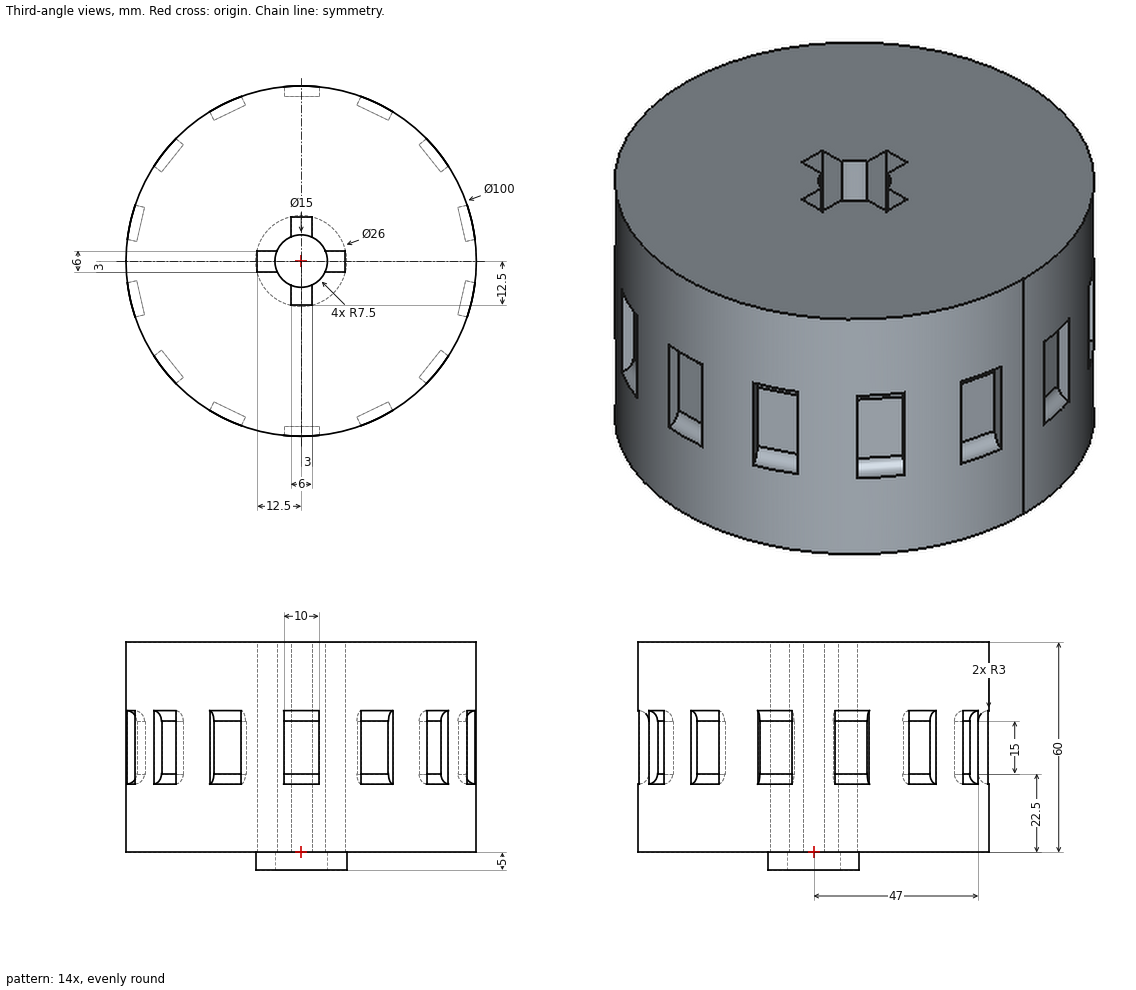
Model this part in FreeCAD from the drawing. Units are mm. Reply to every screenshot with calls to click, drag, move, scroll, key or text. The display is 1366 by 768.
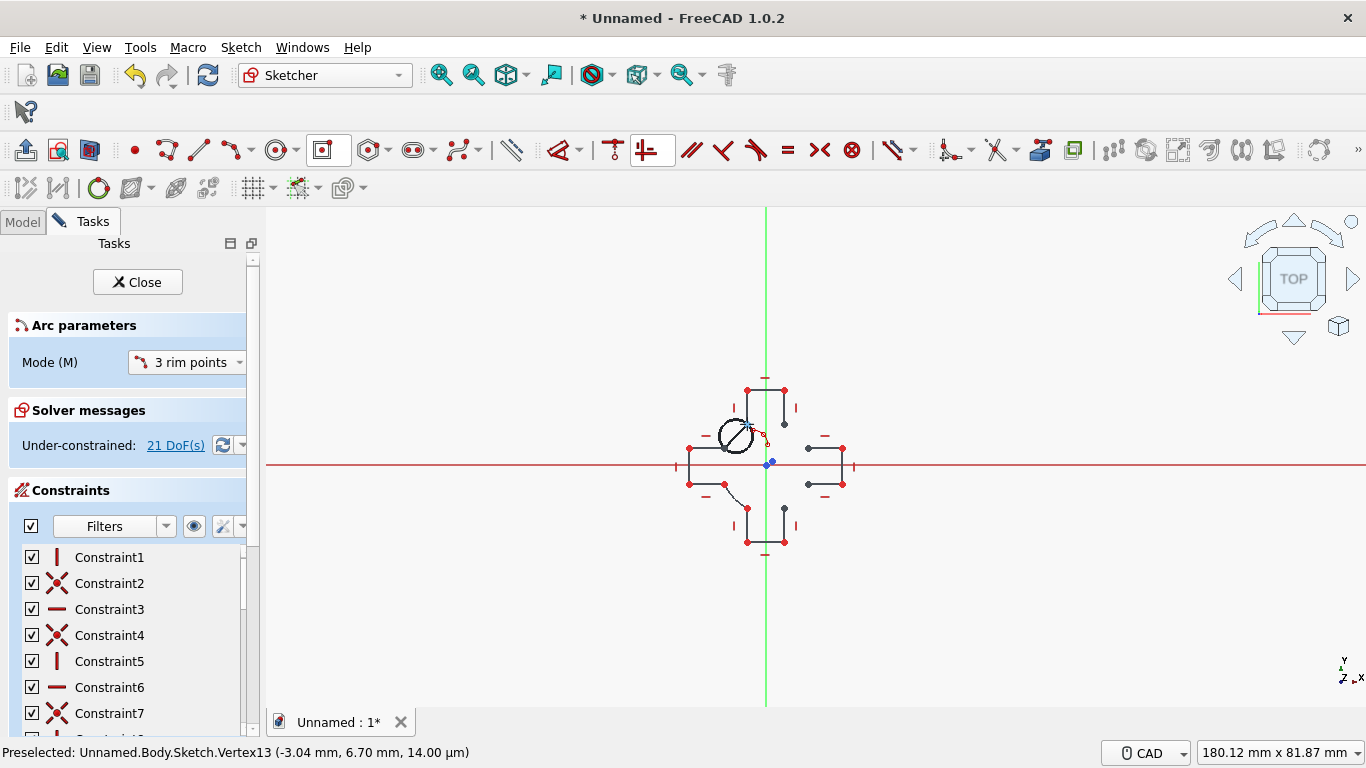
scroll(734, 433, up, 9)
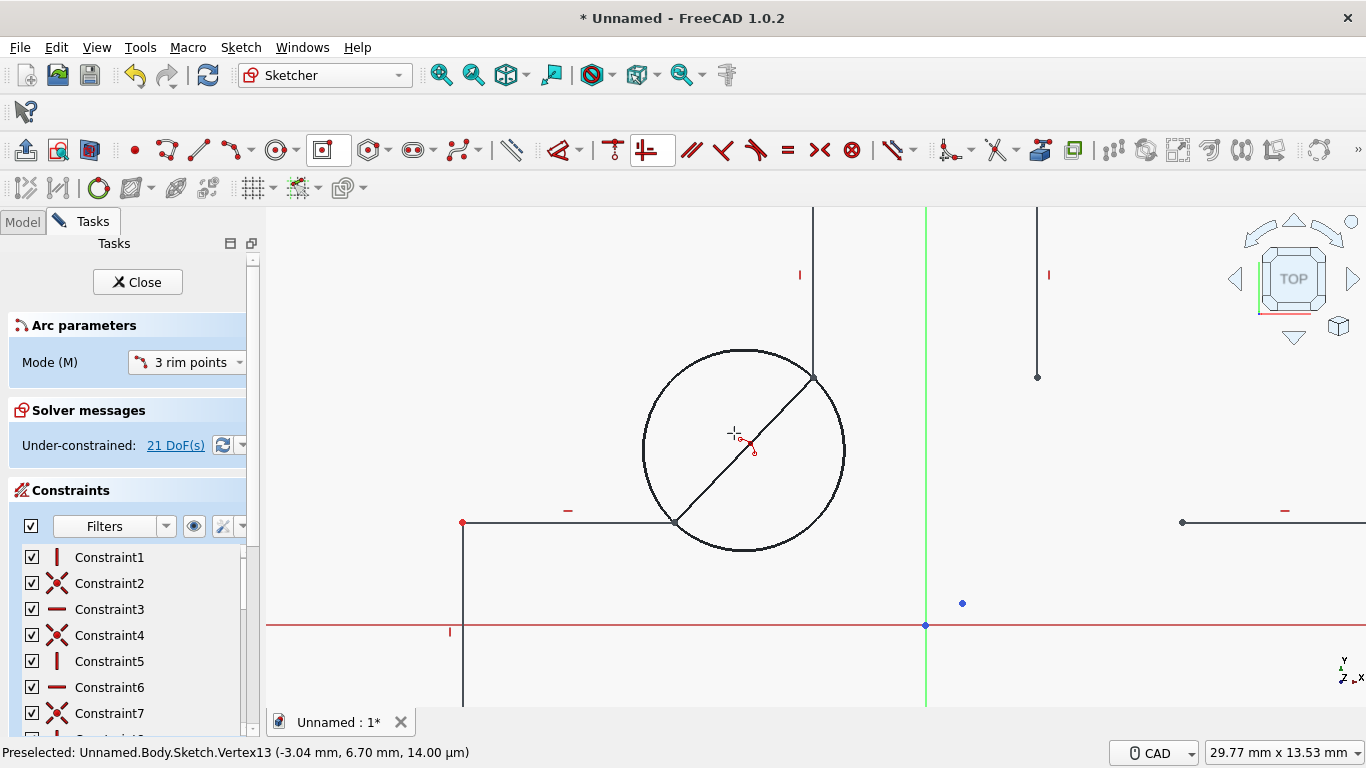
click(730, 430)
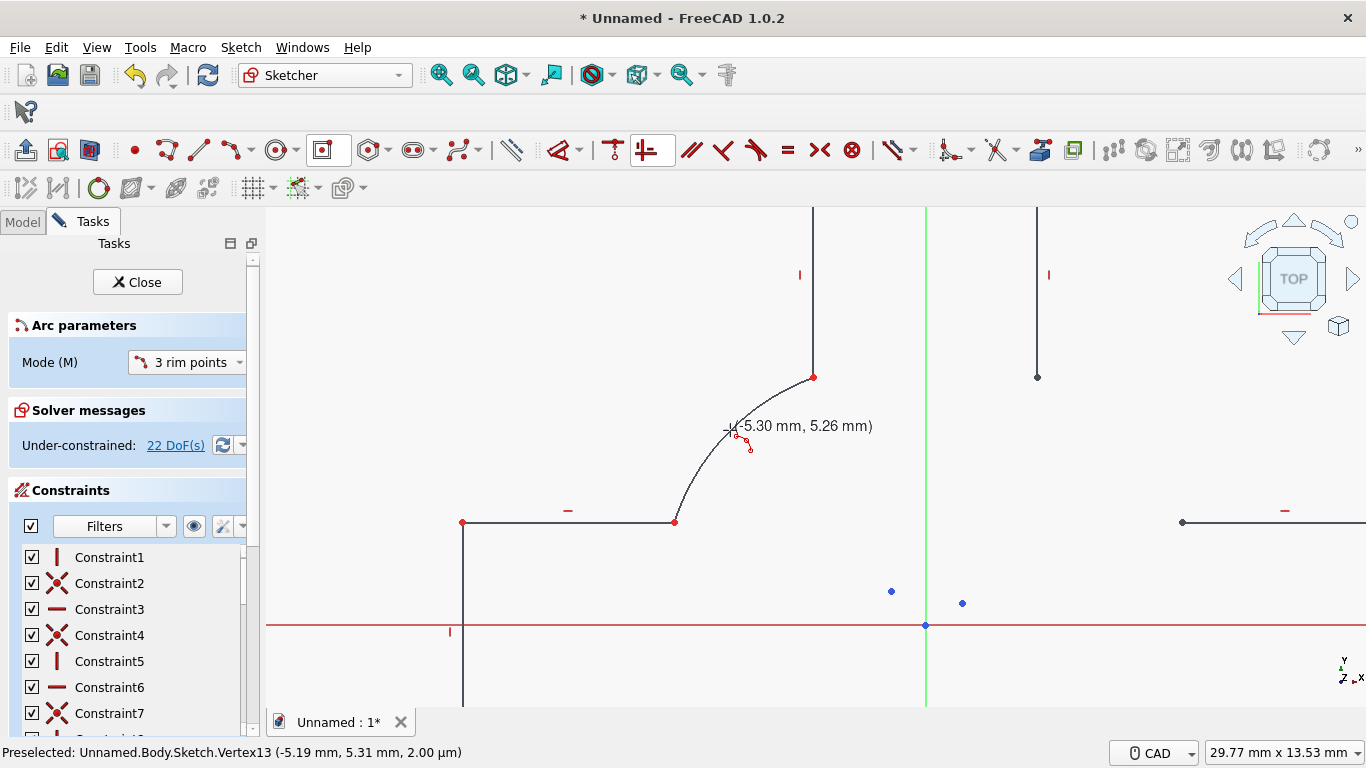
scroll(730, 440, down, 12)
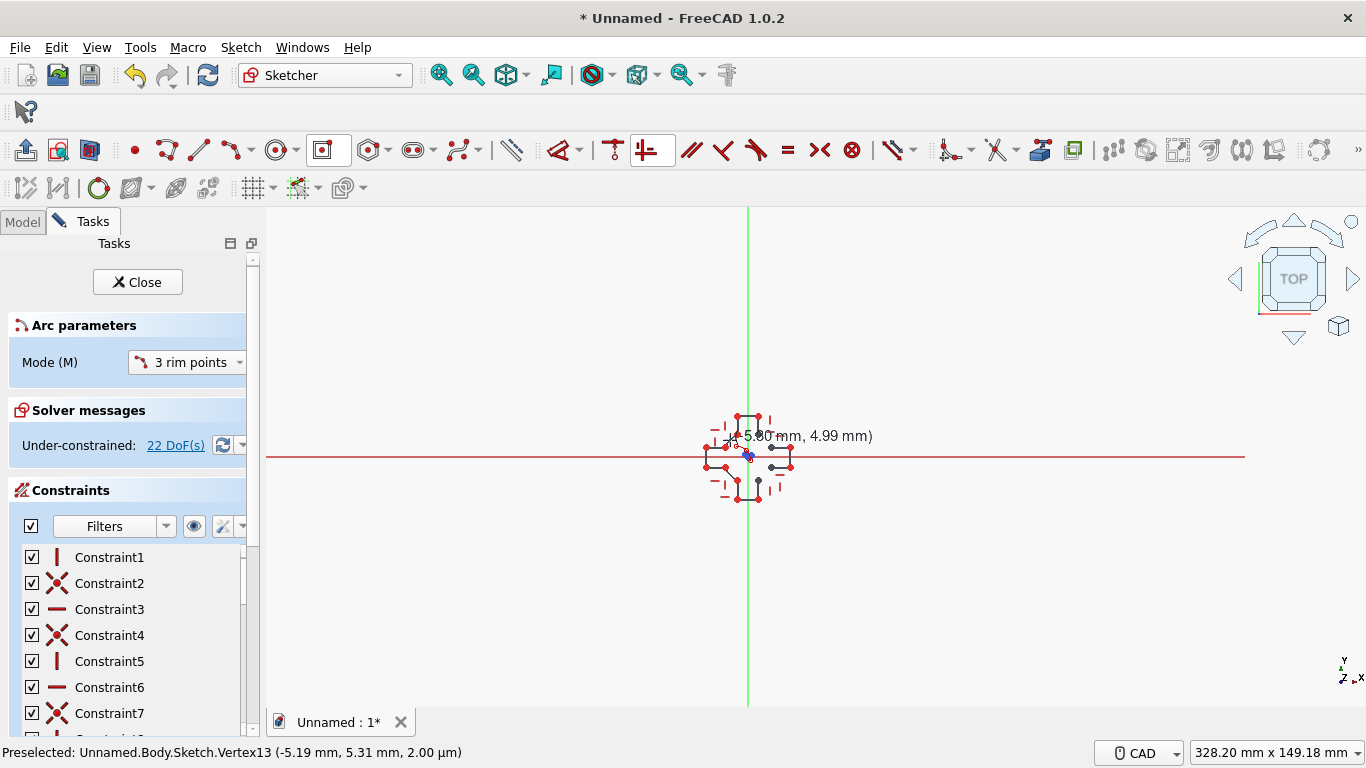
scroll(758, 434, up, 3)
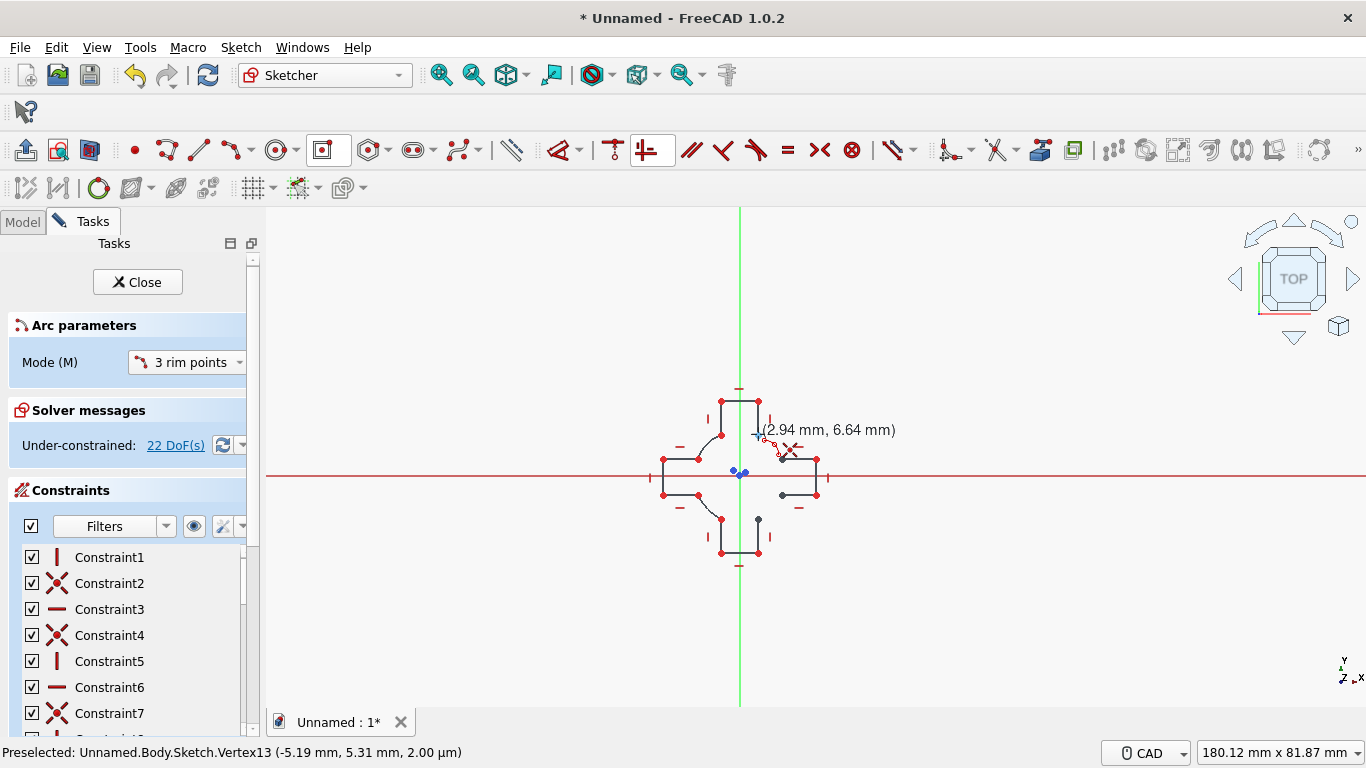
click(758, 435)
click(782, 459)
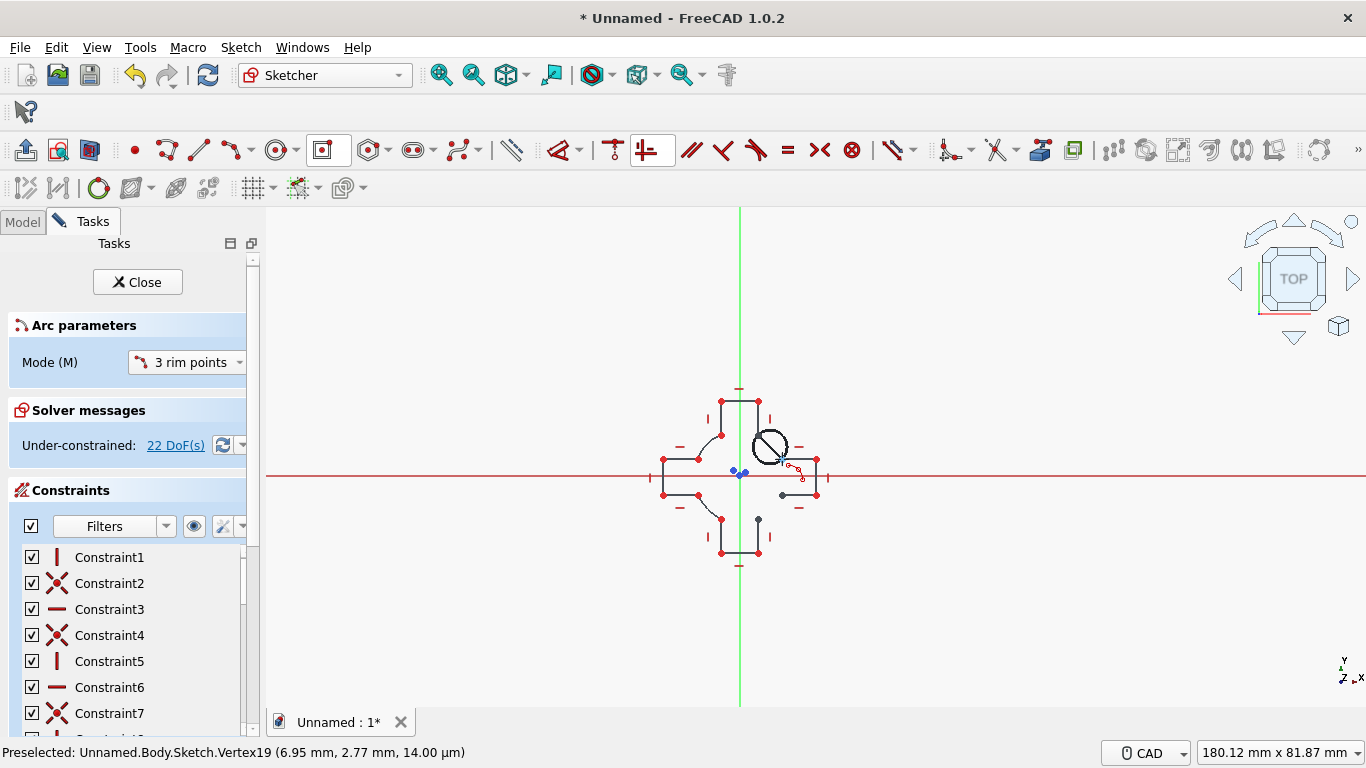
scroll(772, 444, up, 9)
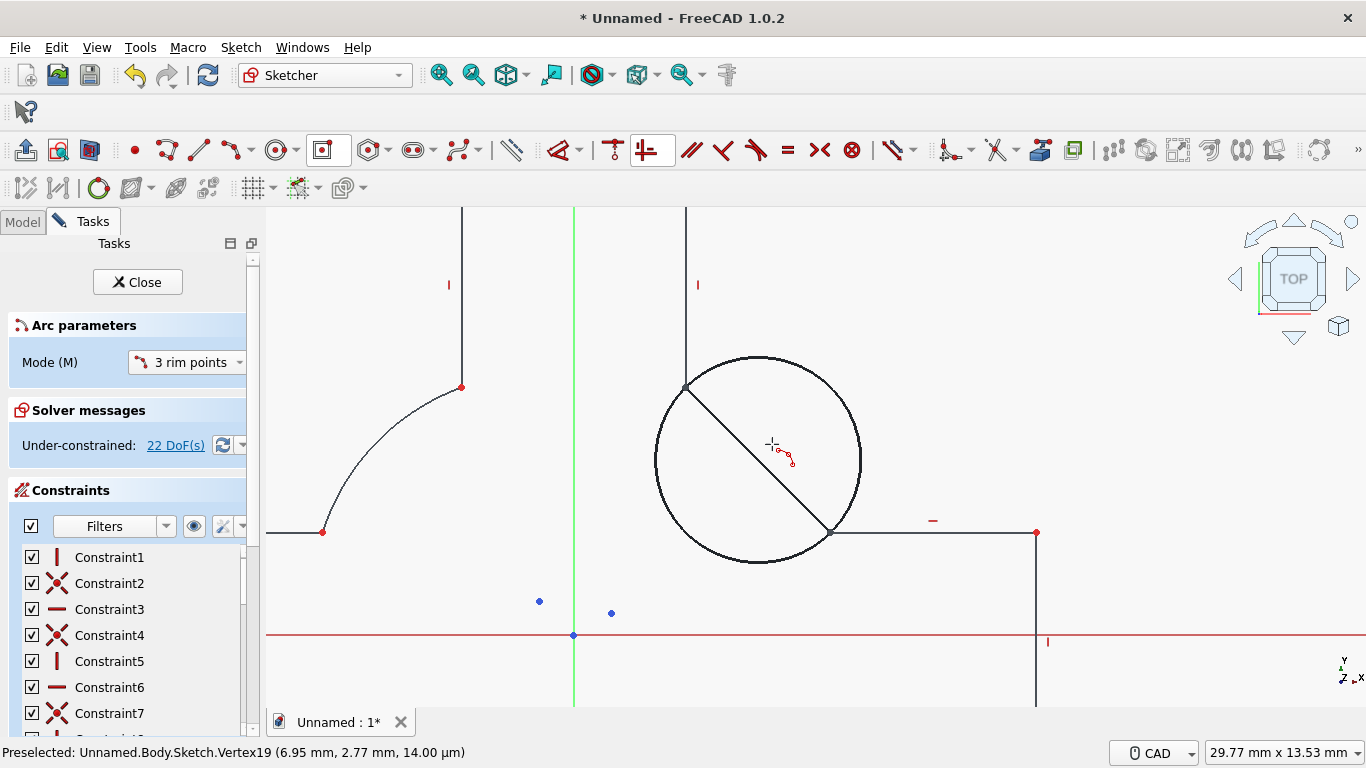
click(770, 439)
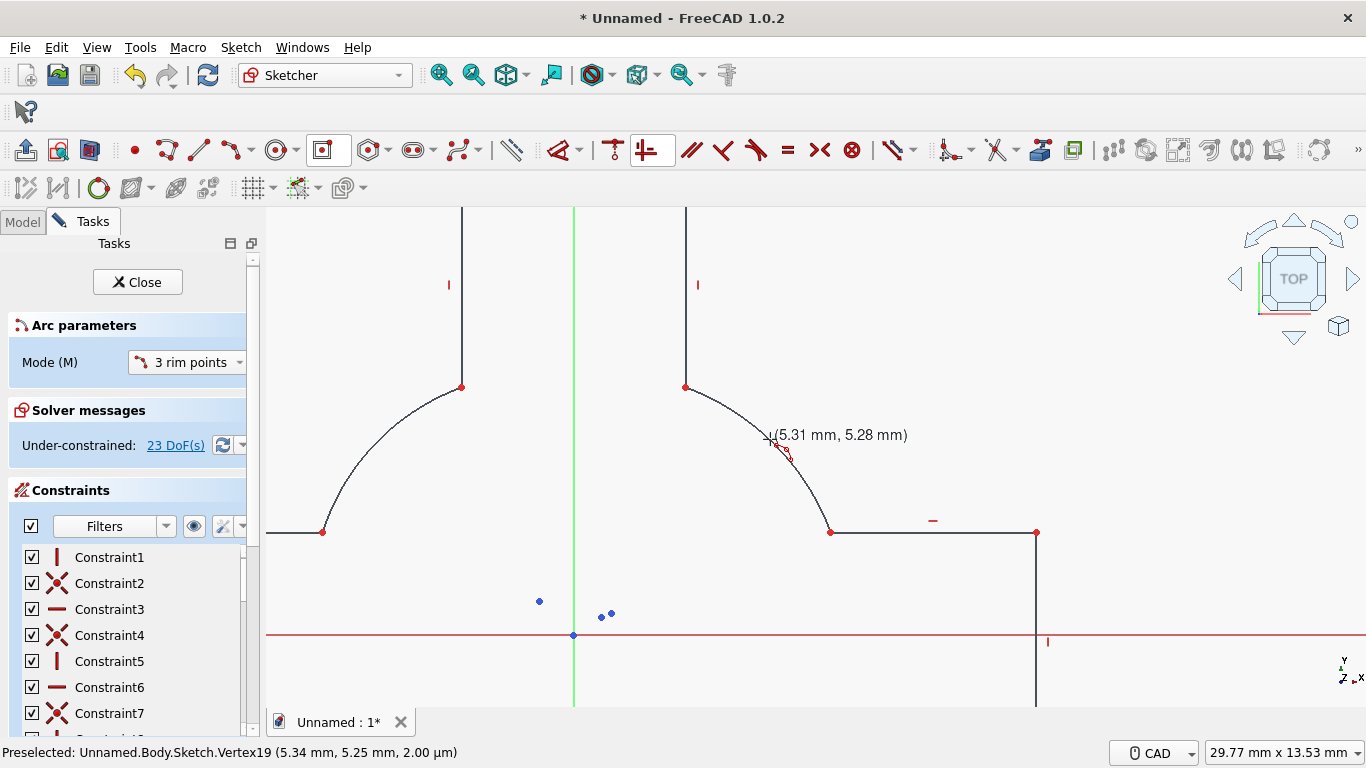
scroll(765, 439, down, 12)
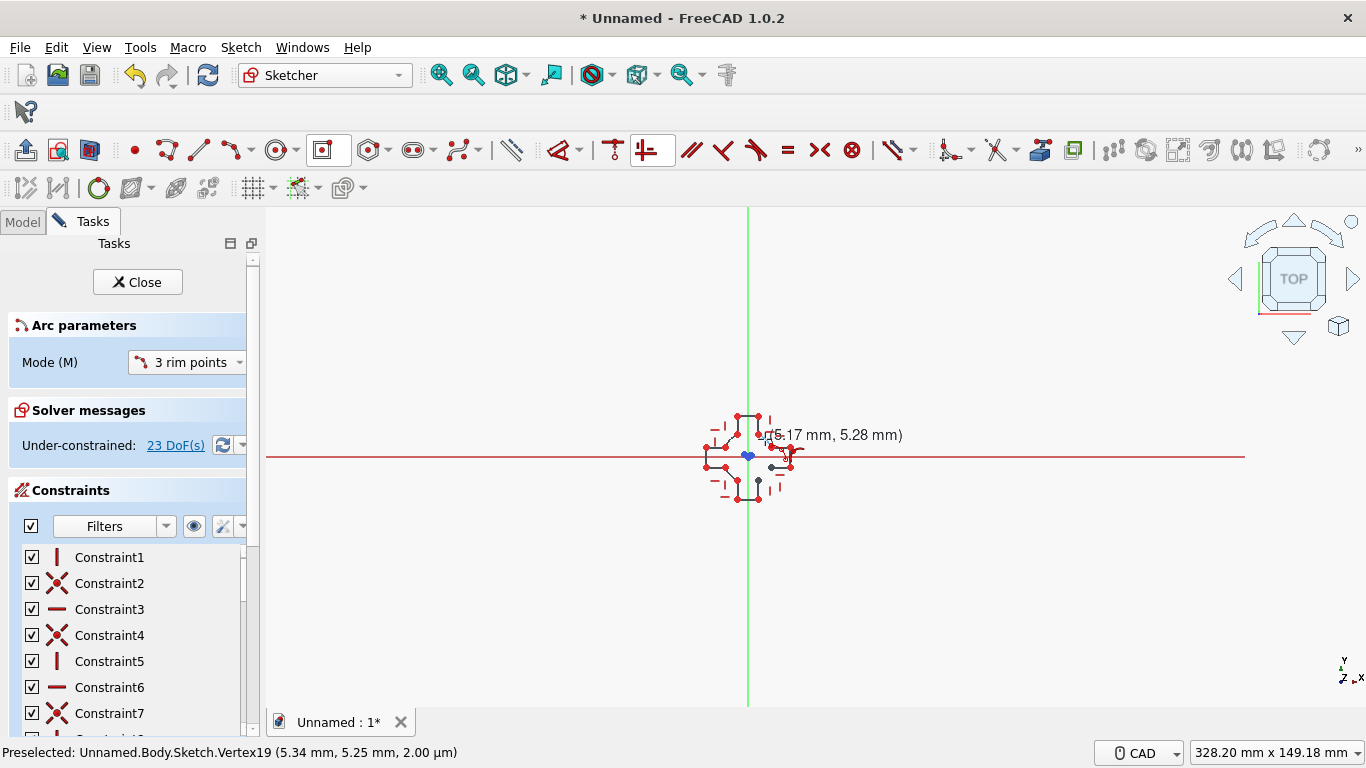
scroll(771, 467, up, 3)